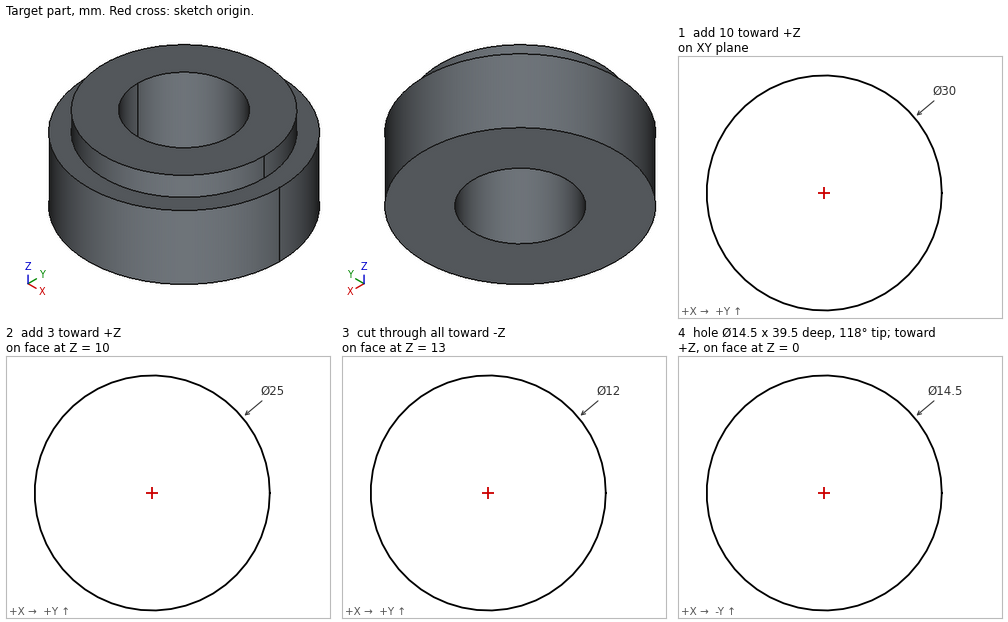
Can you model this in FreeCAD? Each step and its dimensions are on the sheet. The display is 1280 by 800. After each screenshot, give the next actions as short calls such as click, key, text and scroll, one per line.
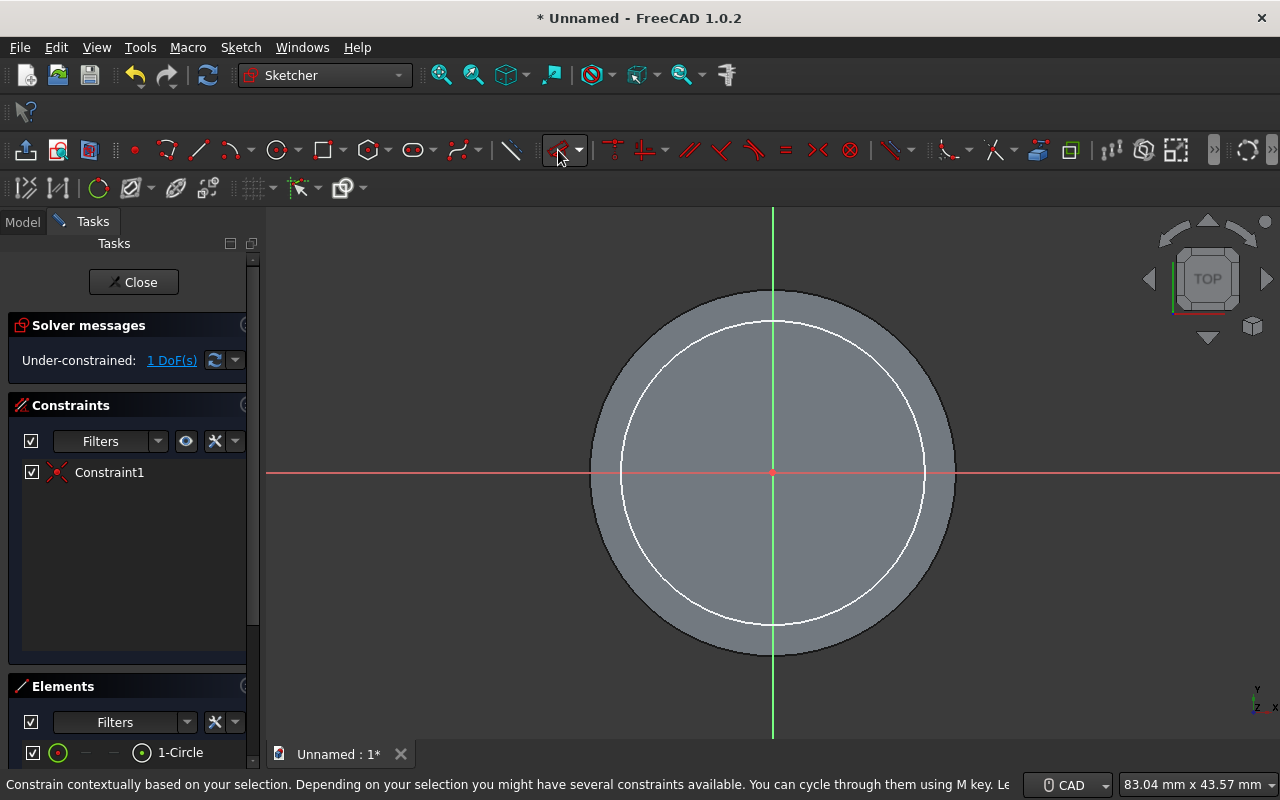
click(880, 365)
click(903, 342)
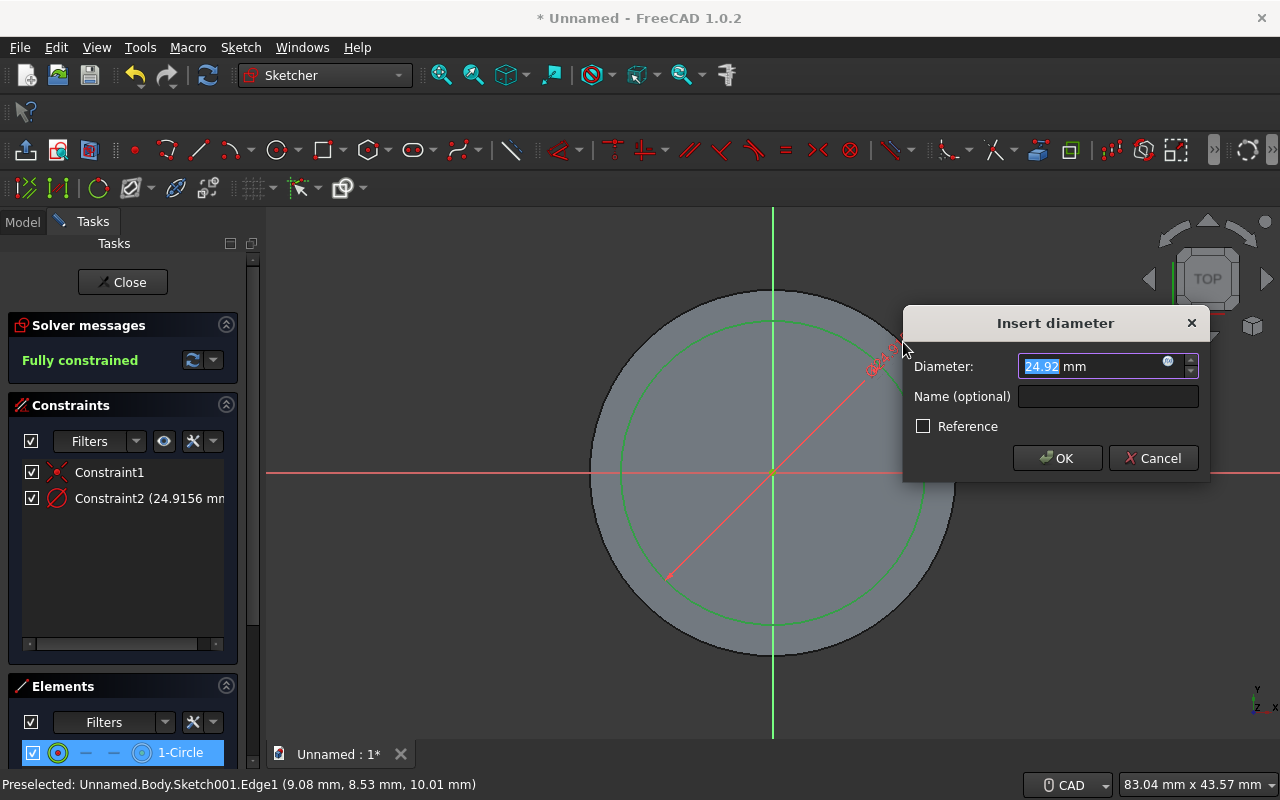
text(25)
key(Return)
key(Escape)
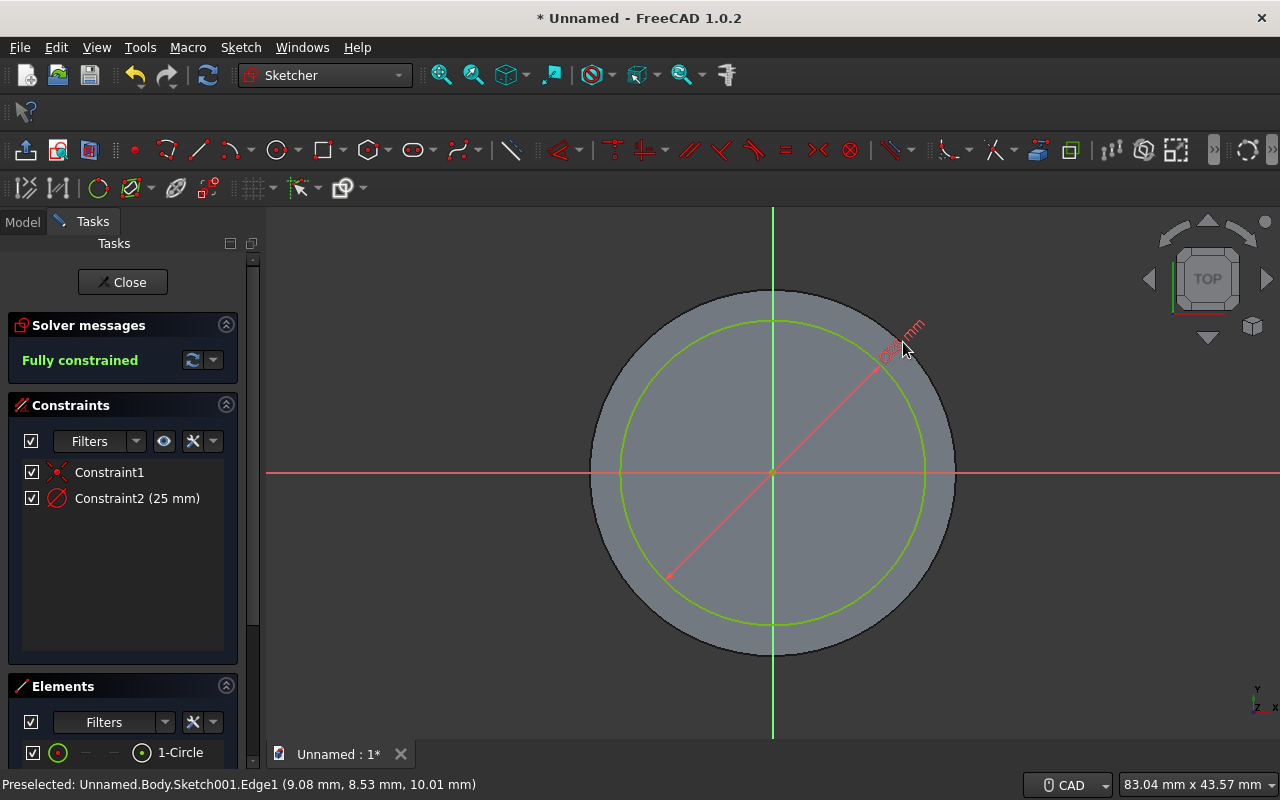
click(123, 282)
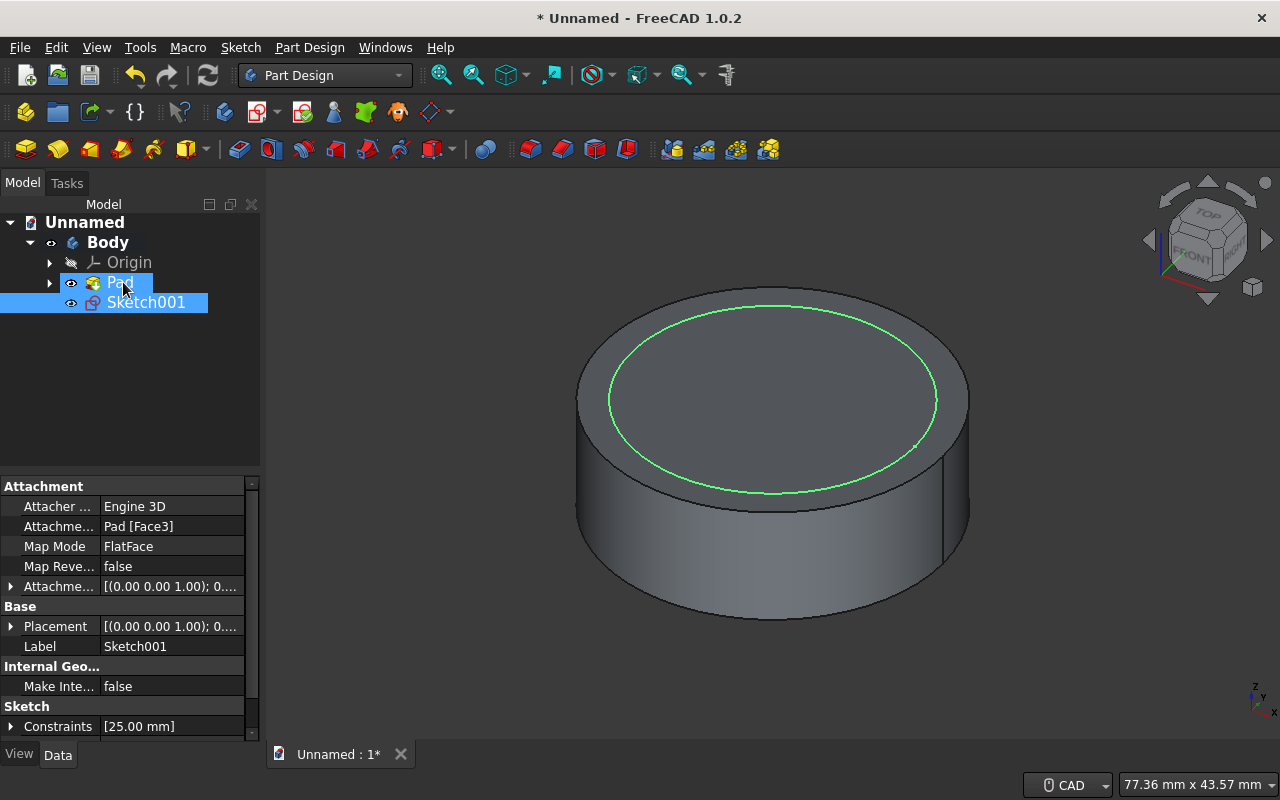
click(26, 150)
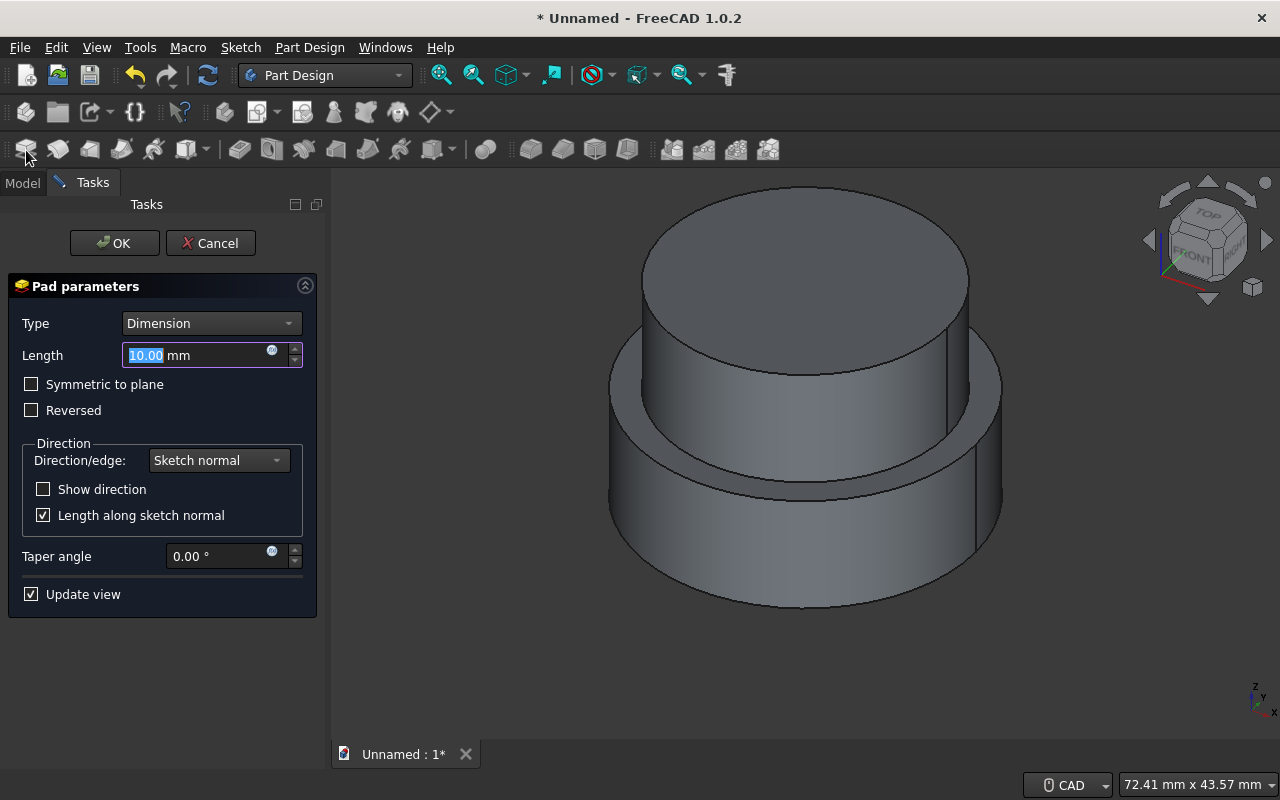
text(3)
key(Tab)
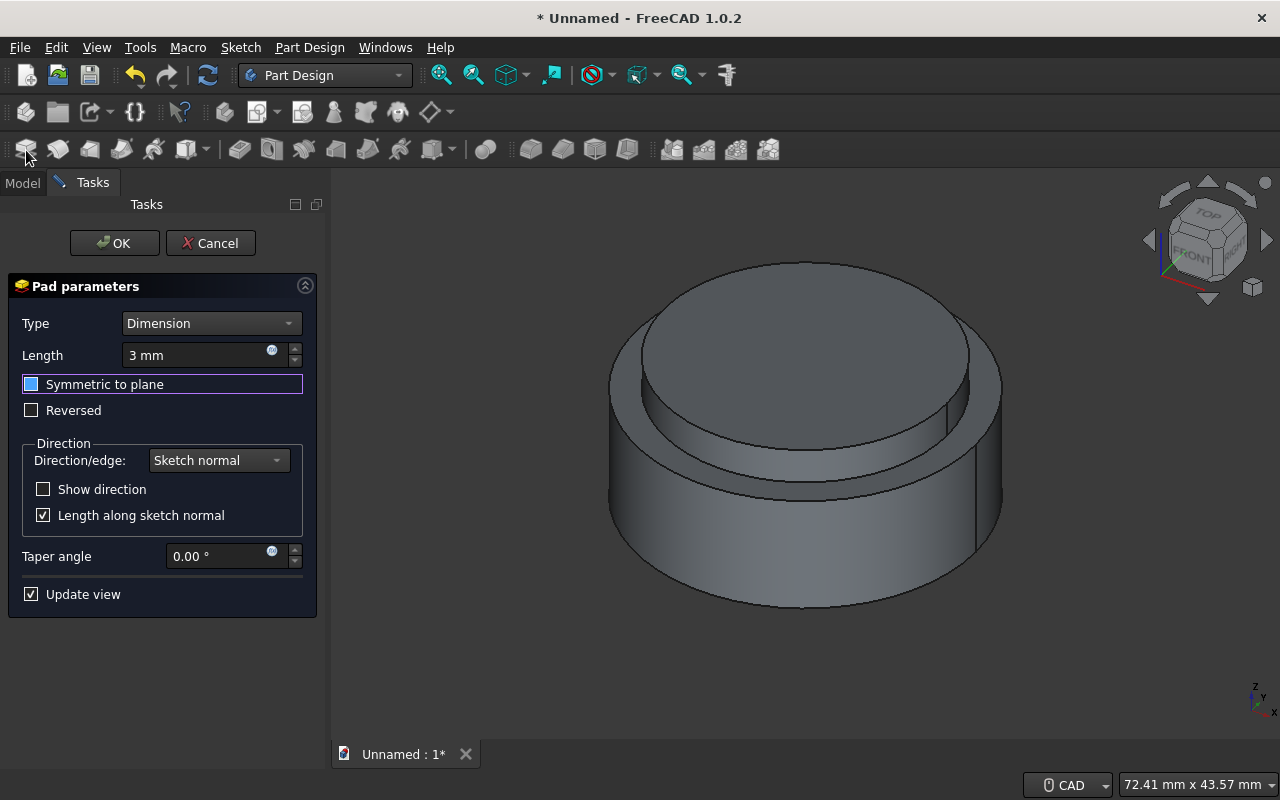
click(115, 243)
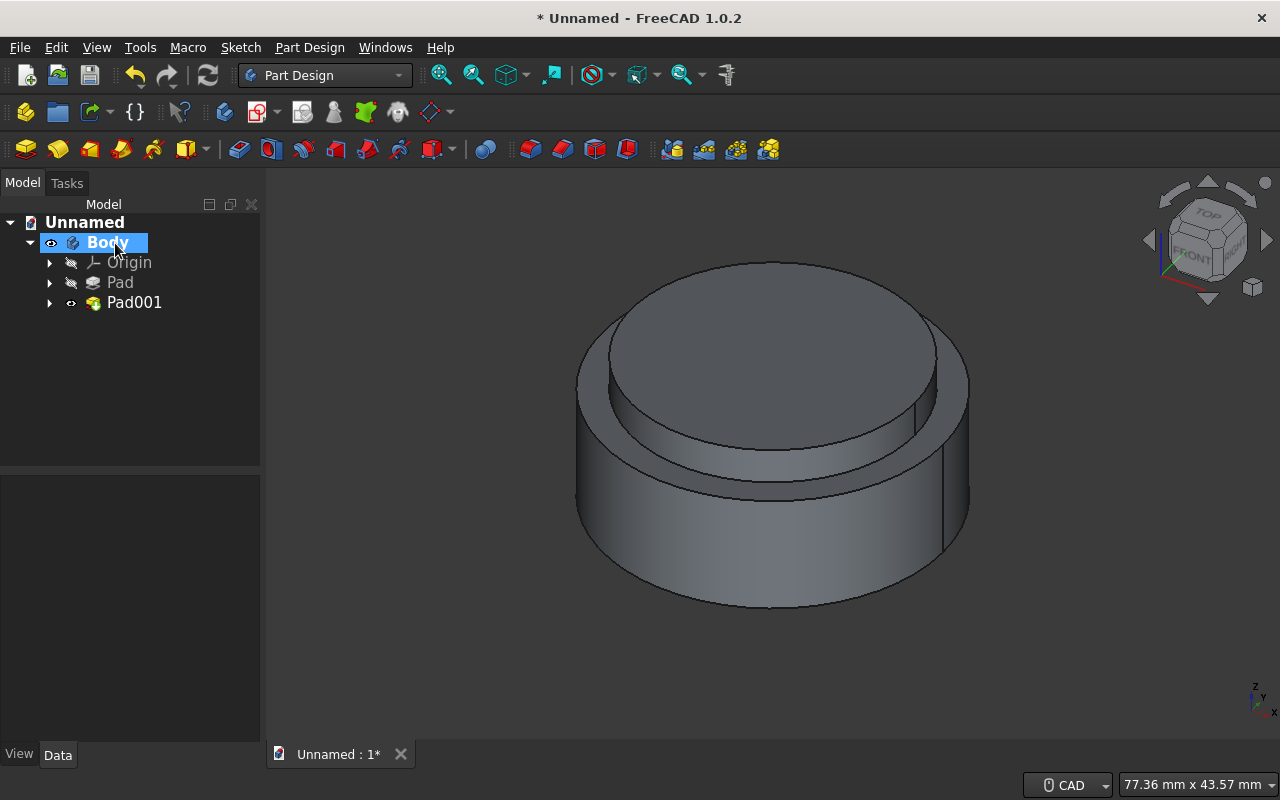
click(773, 355)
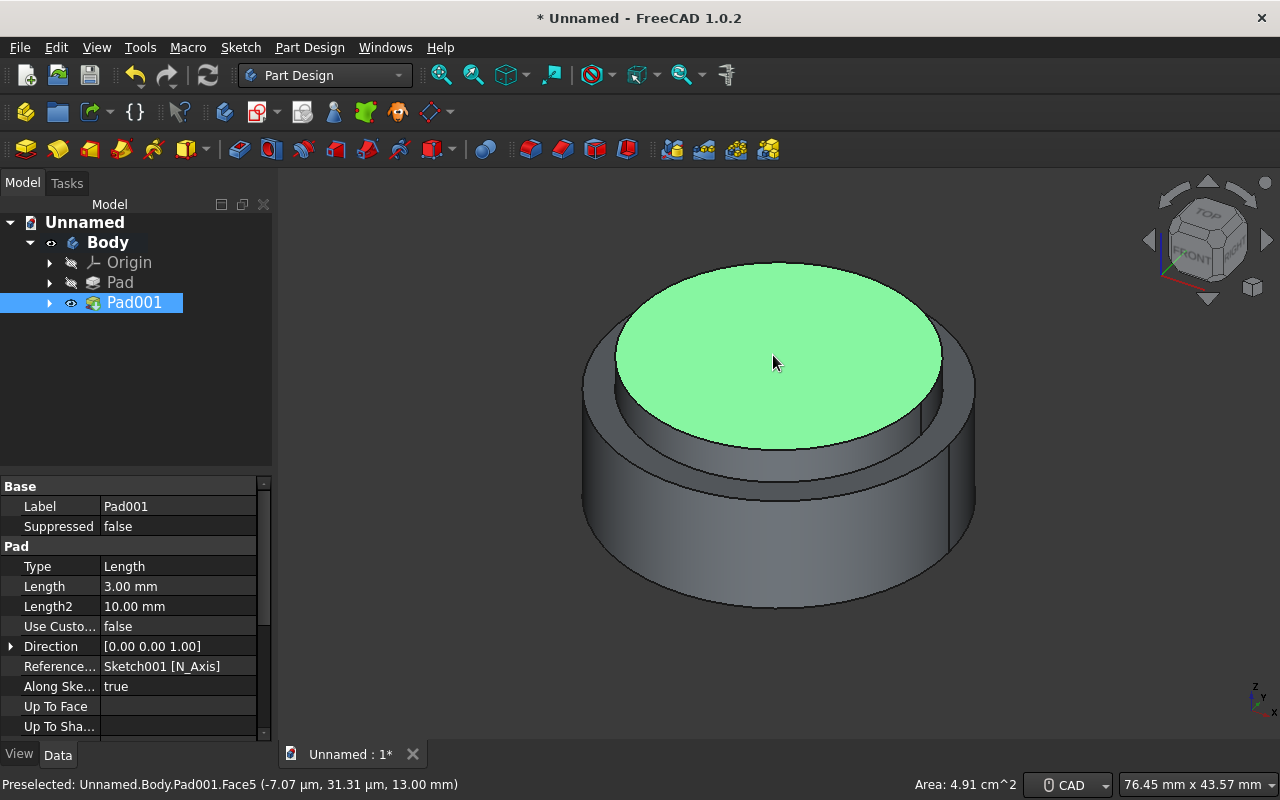
click(258, 112)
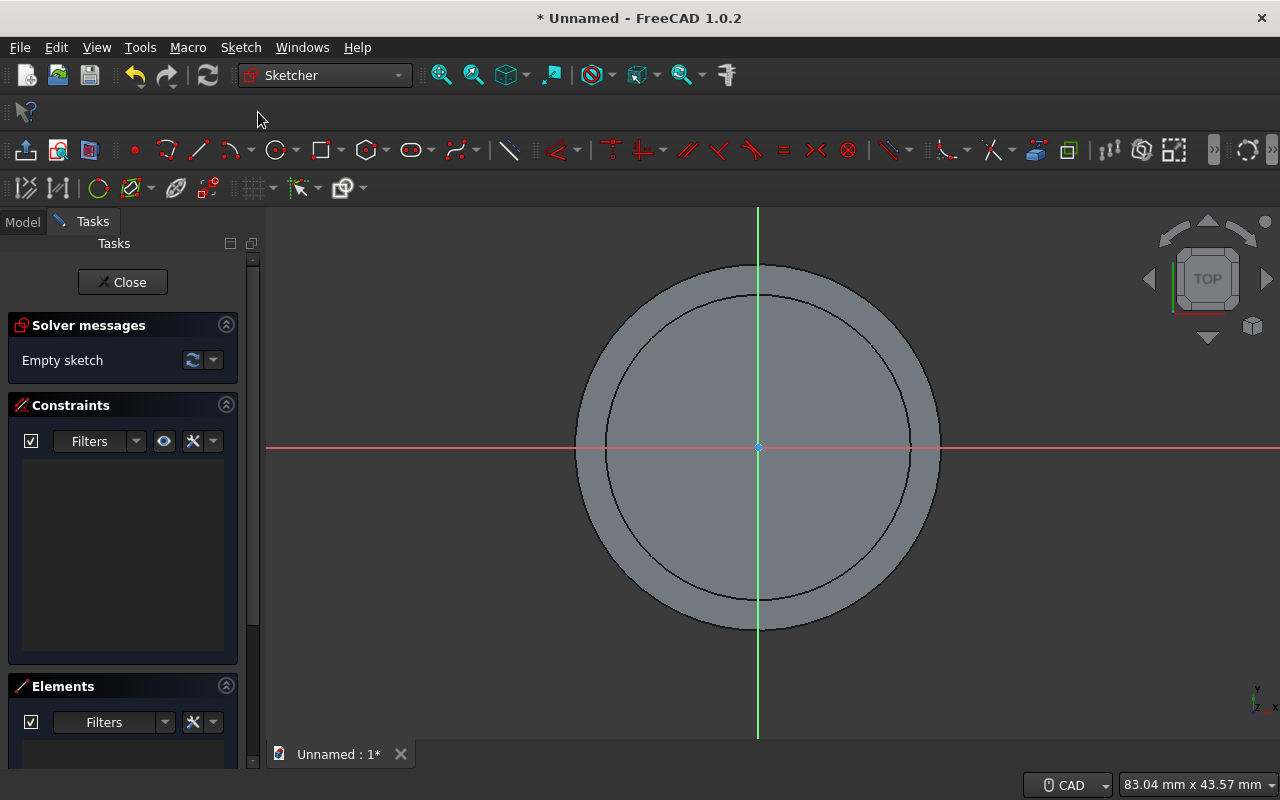
scroll(802, 427, up, 4)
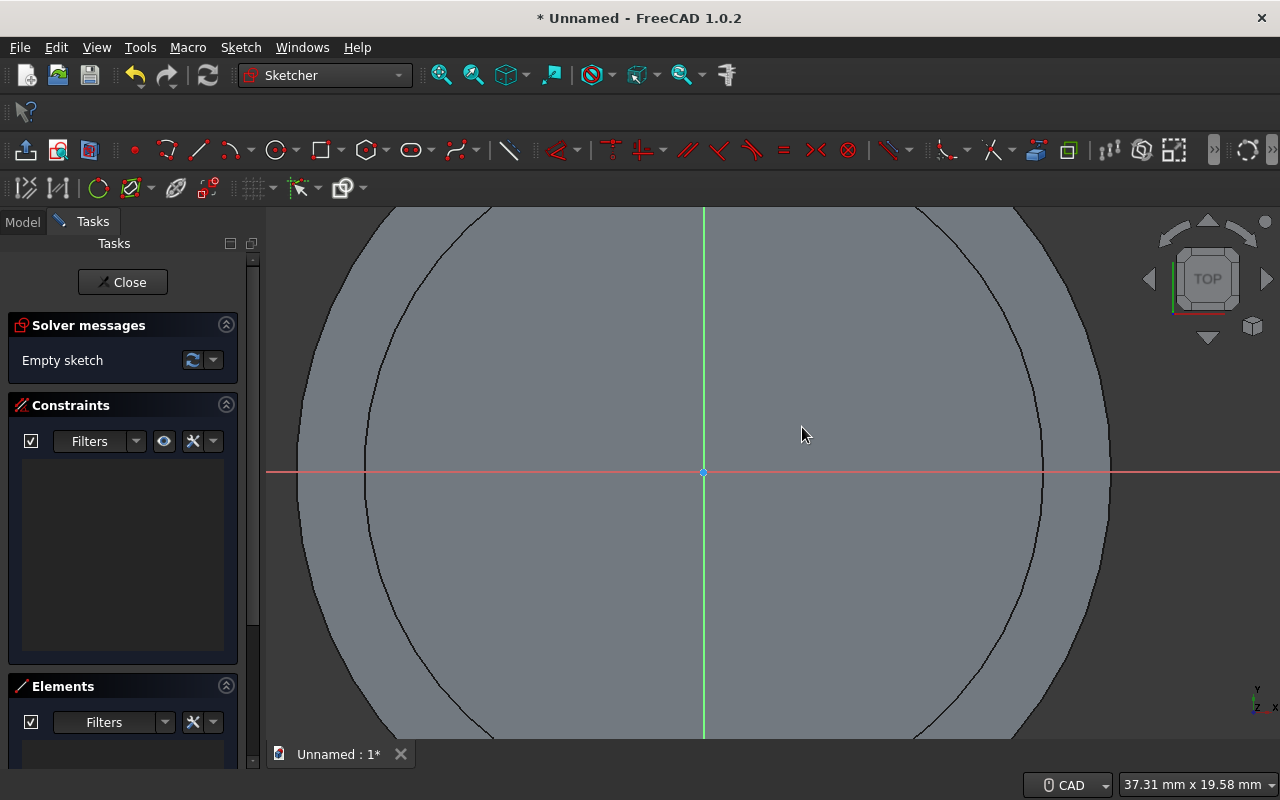
click(276, 150)